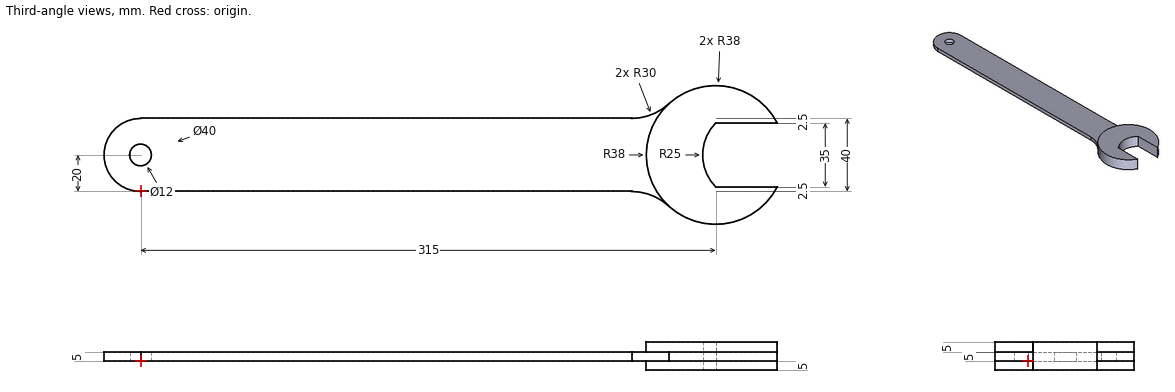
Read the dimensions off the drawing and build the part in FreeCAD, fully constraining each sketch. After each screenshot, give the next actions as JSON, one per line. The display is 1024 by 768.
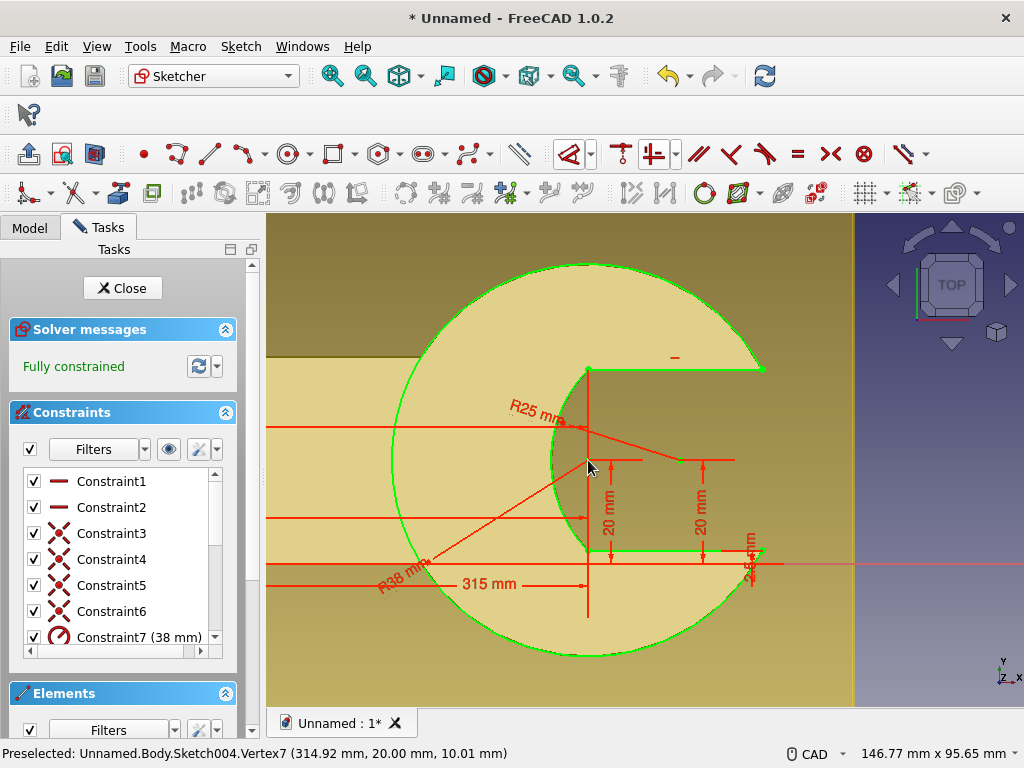
{"action": "left_click", "coordinate": [123, 288]}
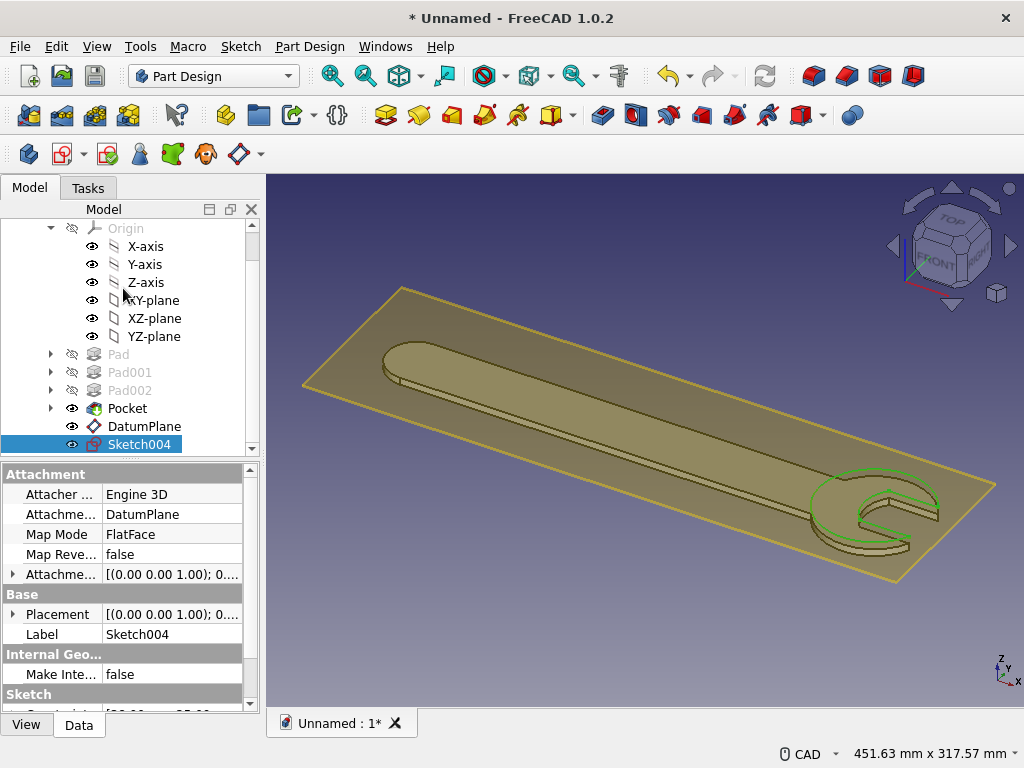
{"action": "left_click", "coordinate": [386, 116]}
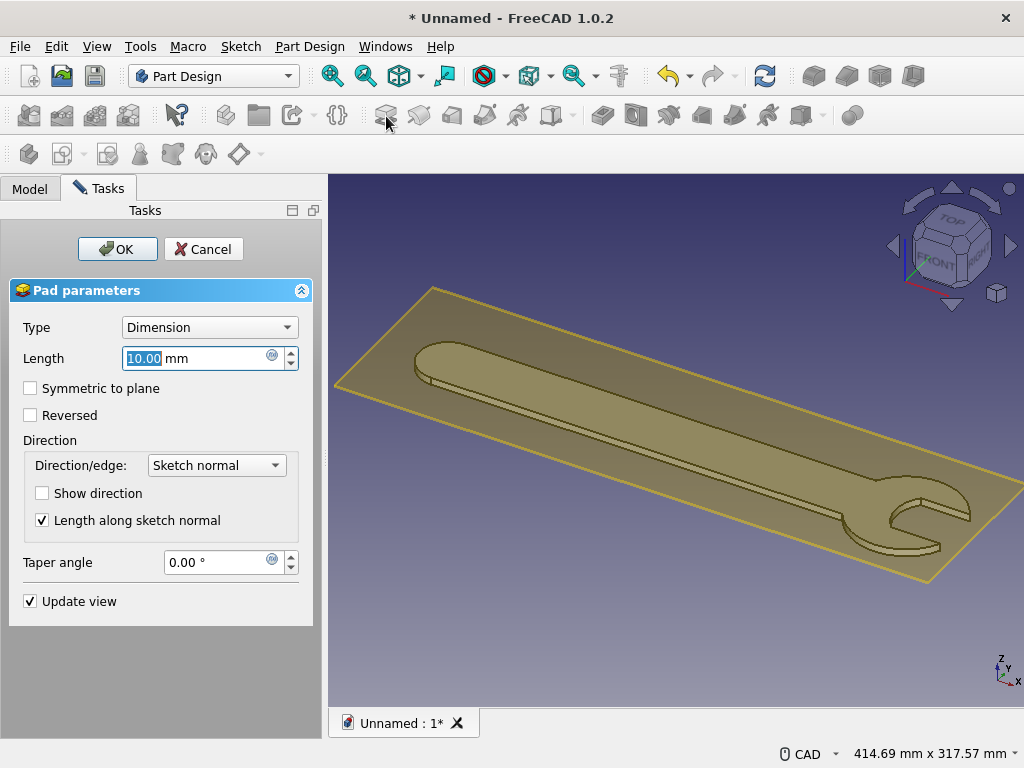
{"action": "type", "text": "5"}
{"action": "key", "text": "Tab"}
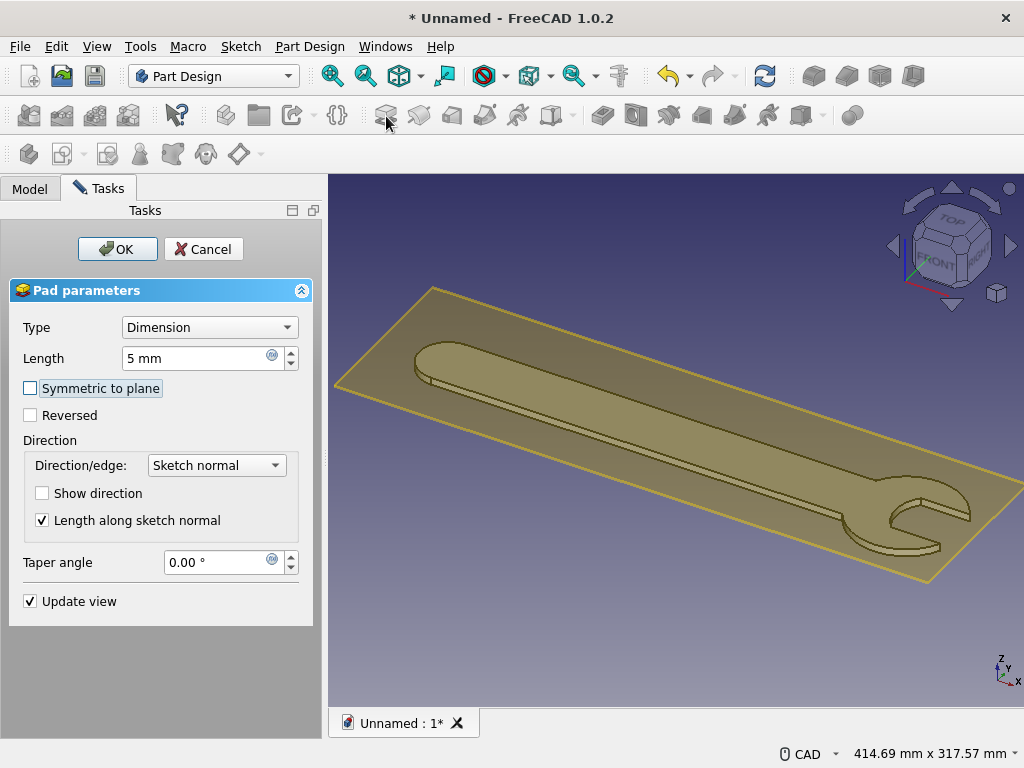
{"action": "left_click", "coordinate": [31, 415]}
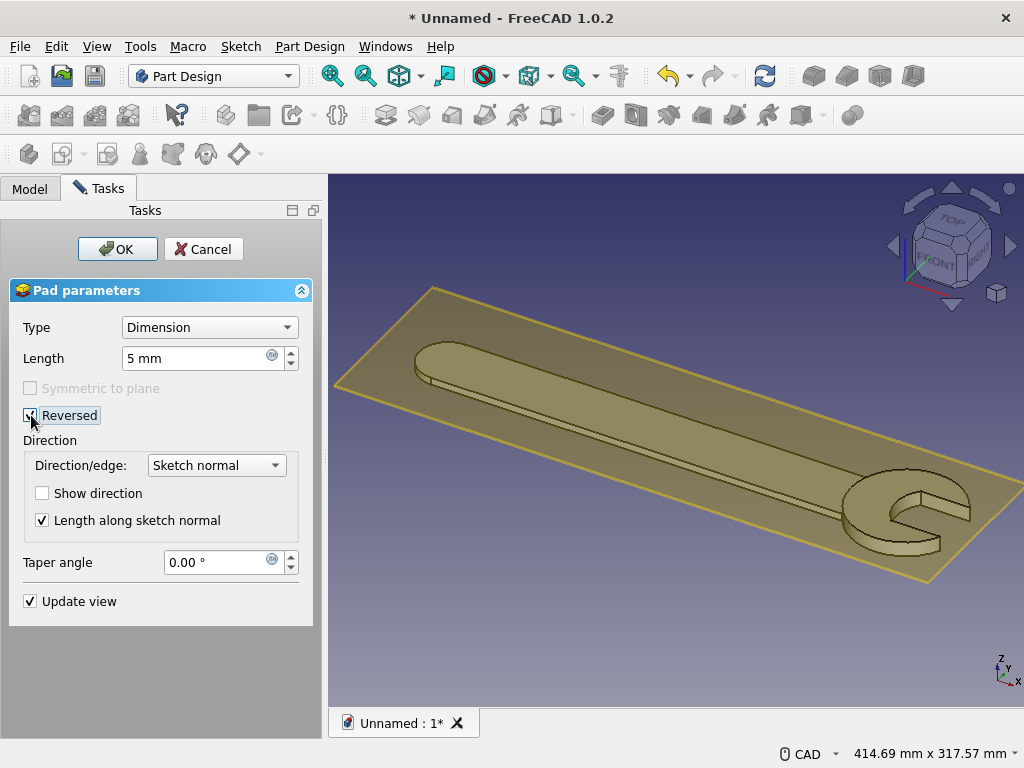
{"action": "left_click", "coordinate": [118, 249]}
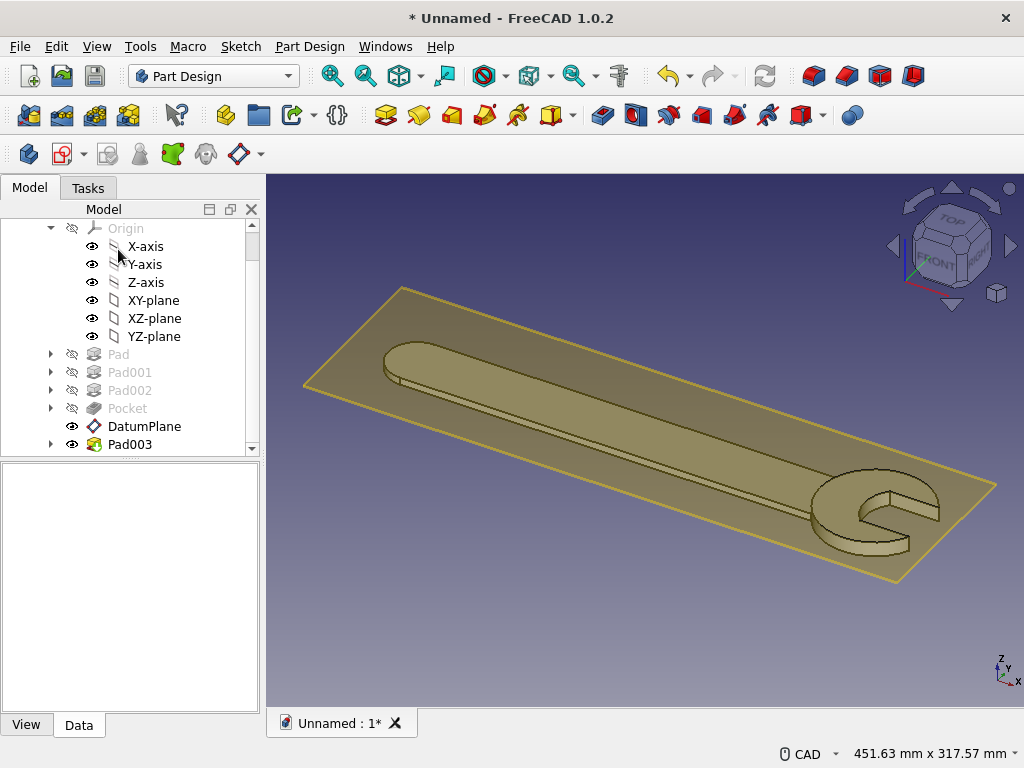
{"action": "left_click", "coordinate": [117, 426]}
{"action": "key", "text": "space"}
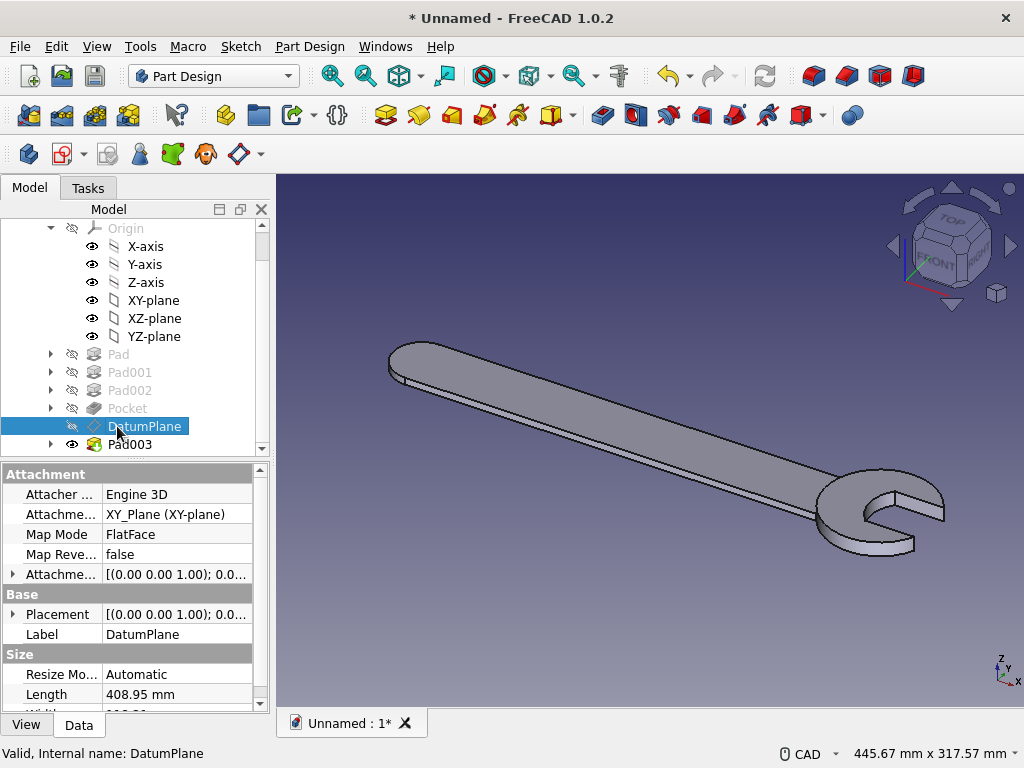
{"action": "left_click", "coordinate": [316, 667]}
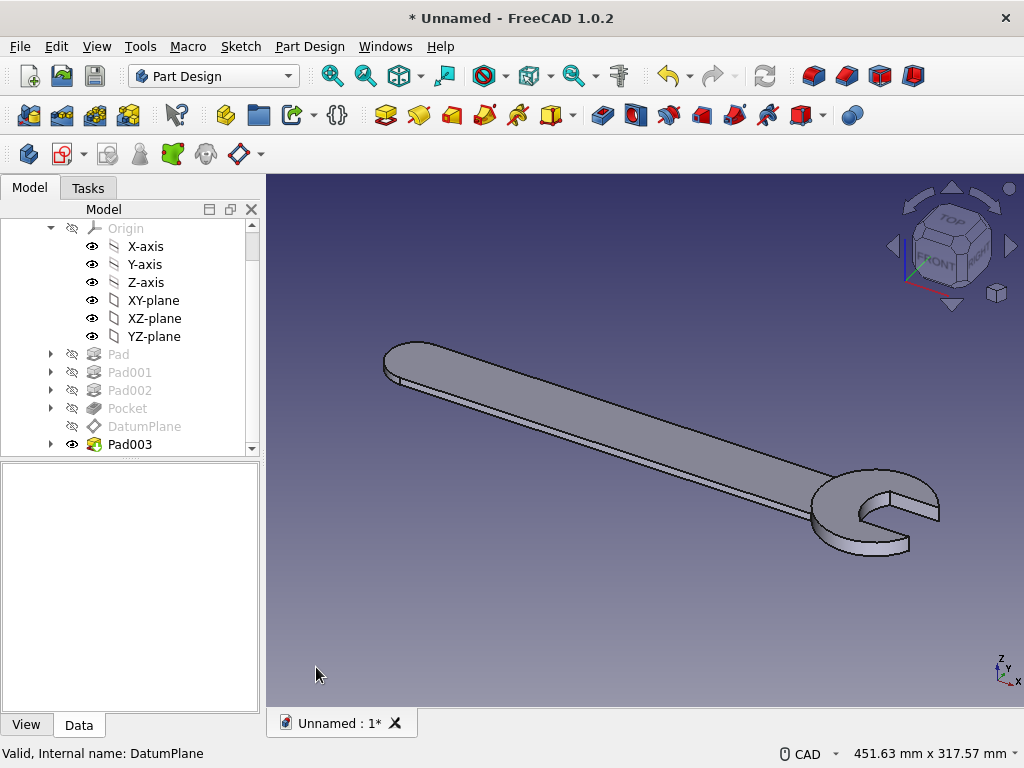
{"action": "left_click", "coordinate": [62, 154]}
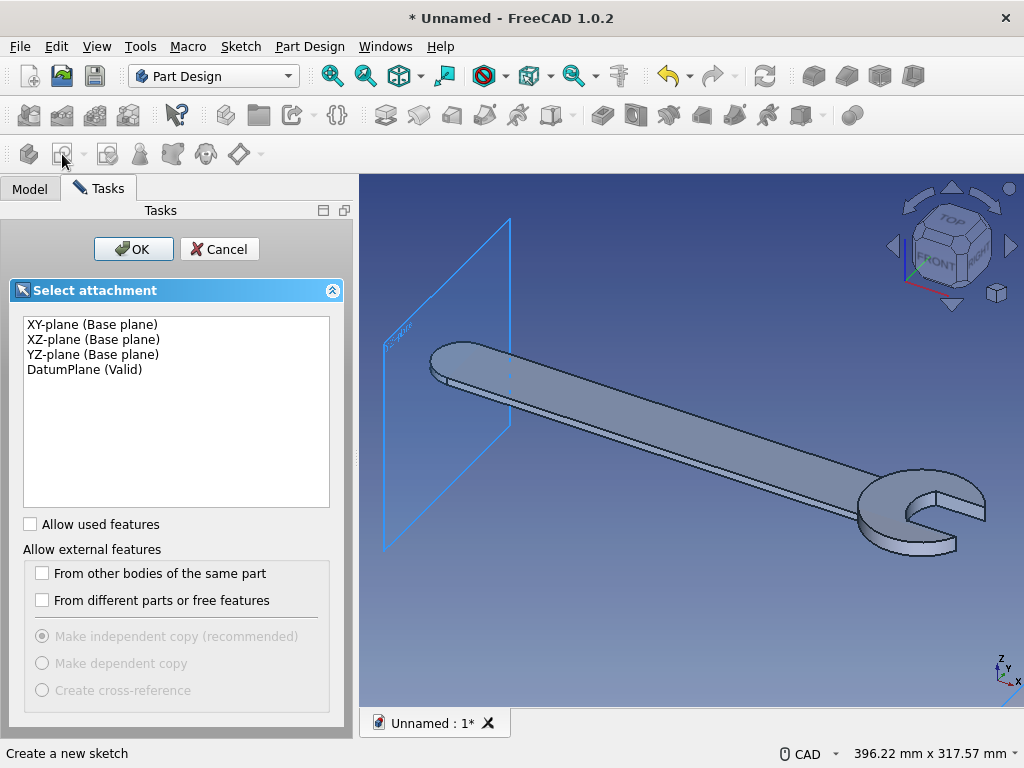
{"action": "left_click", "coordinate": [84, 324]}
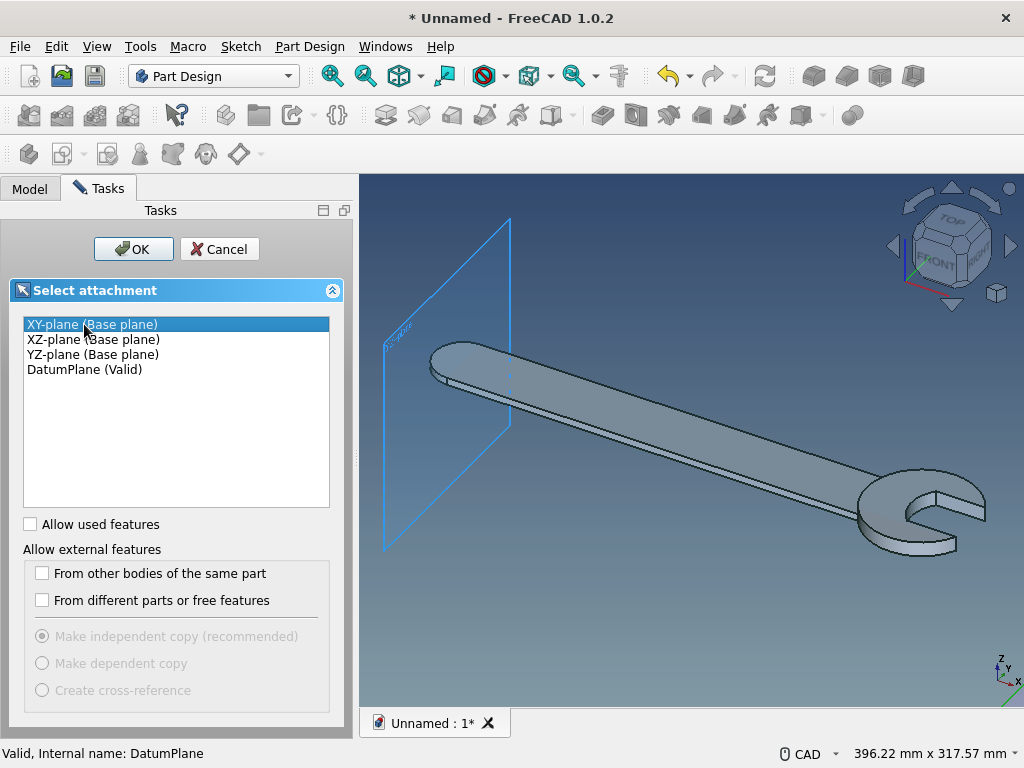
{"action": "left_click", "coordinate": [134, 249]}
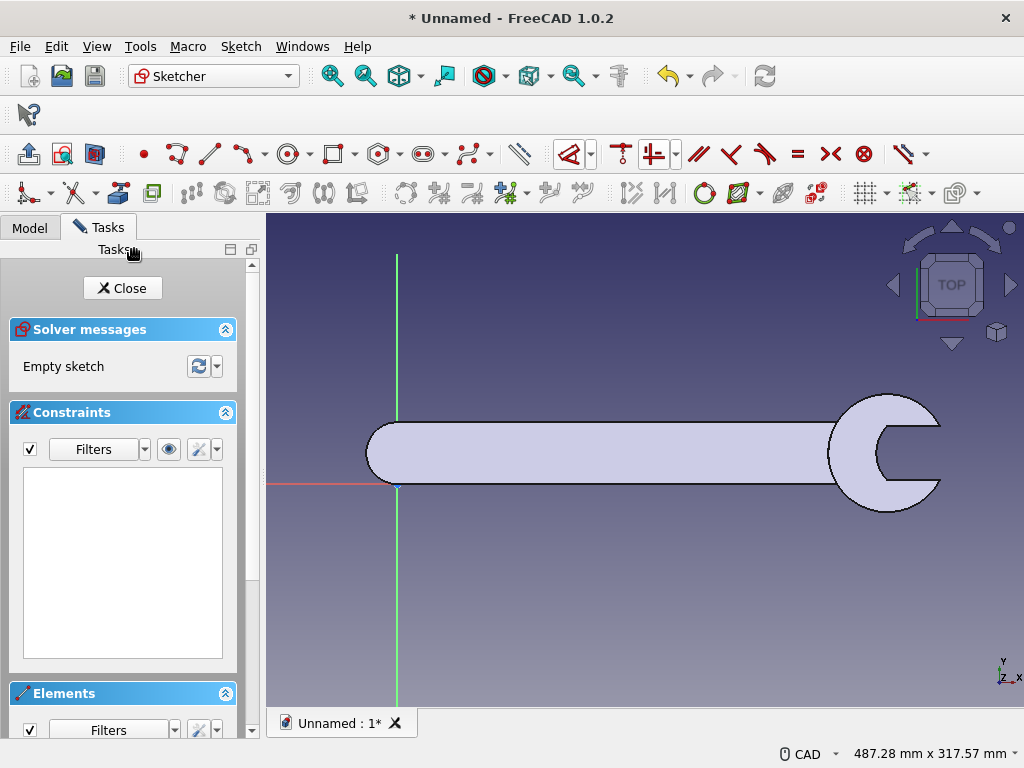
{"action": "left_click", "coordinate": [95, 154]}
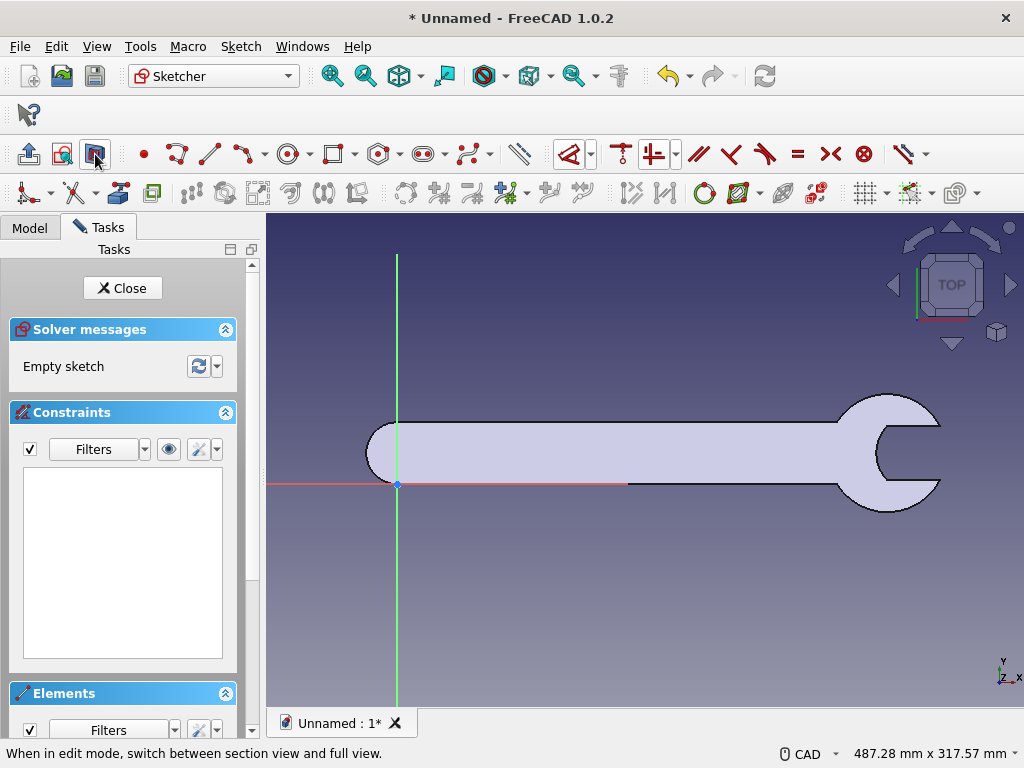
{"action": "scroll", "coordinate": [576, 460], "scroll_direction": "down", "scroll_amount": 5}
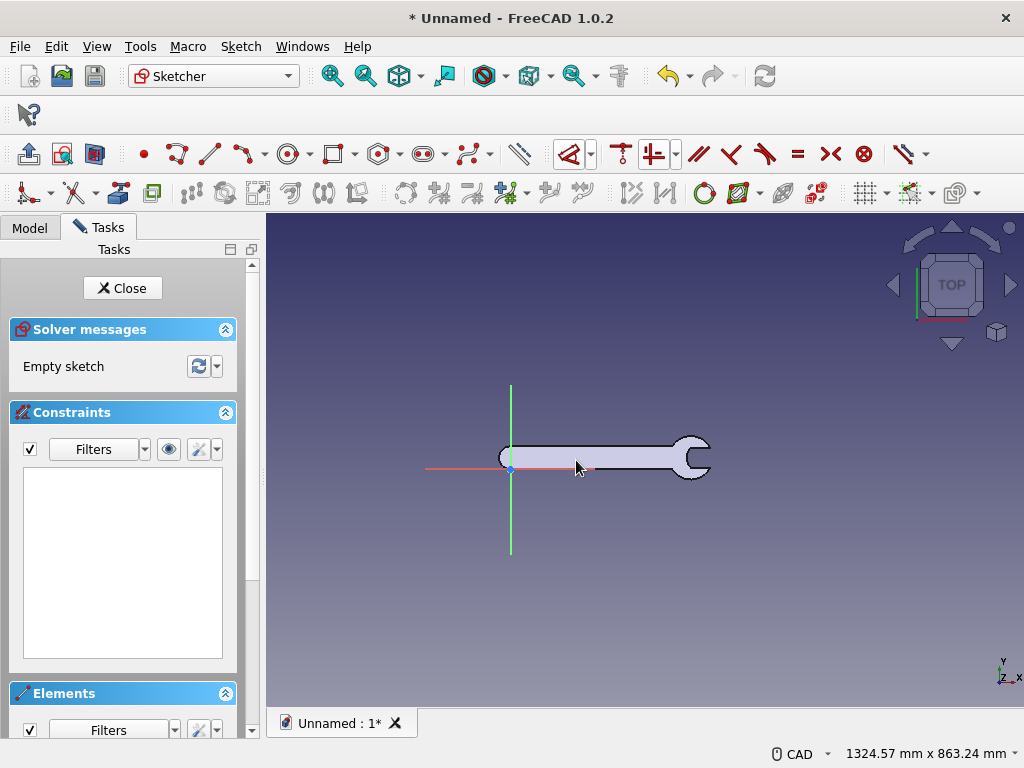
{"action": "scroll", "coordinate": [704, 458], "scroll_direction": "up", "scroll_amount": 11}